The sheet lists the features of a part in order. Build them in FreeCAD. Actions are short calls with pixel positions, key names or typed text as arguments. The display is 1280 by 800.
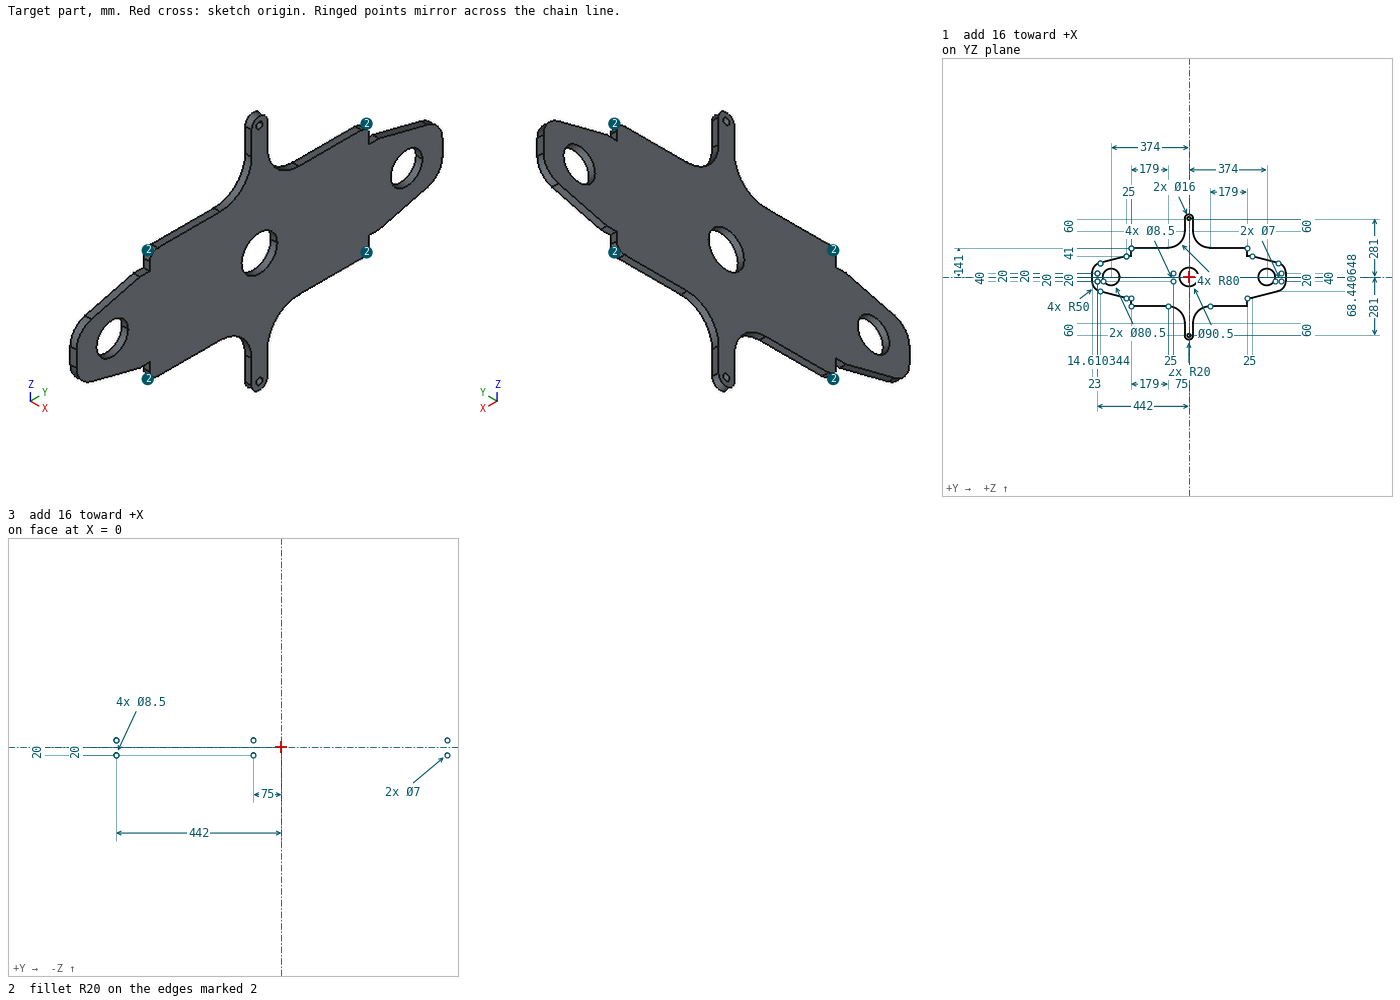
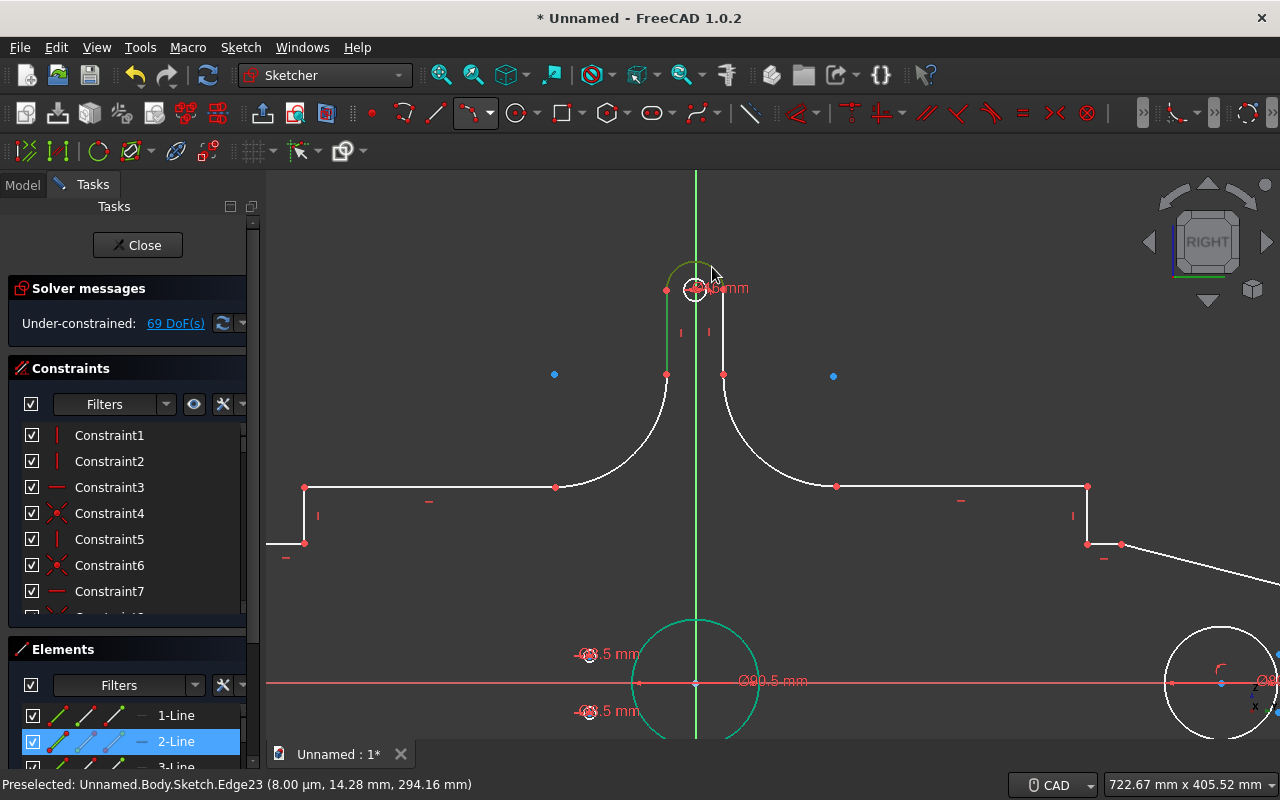
click(992, 114)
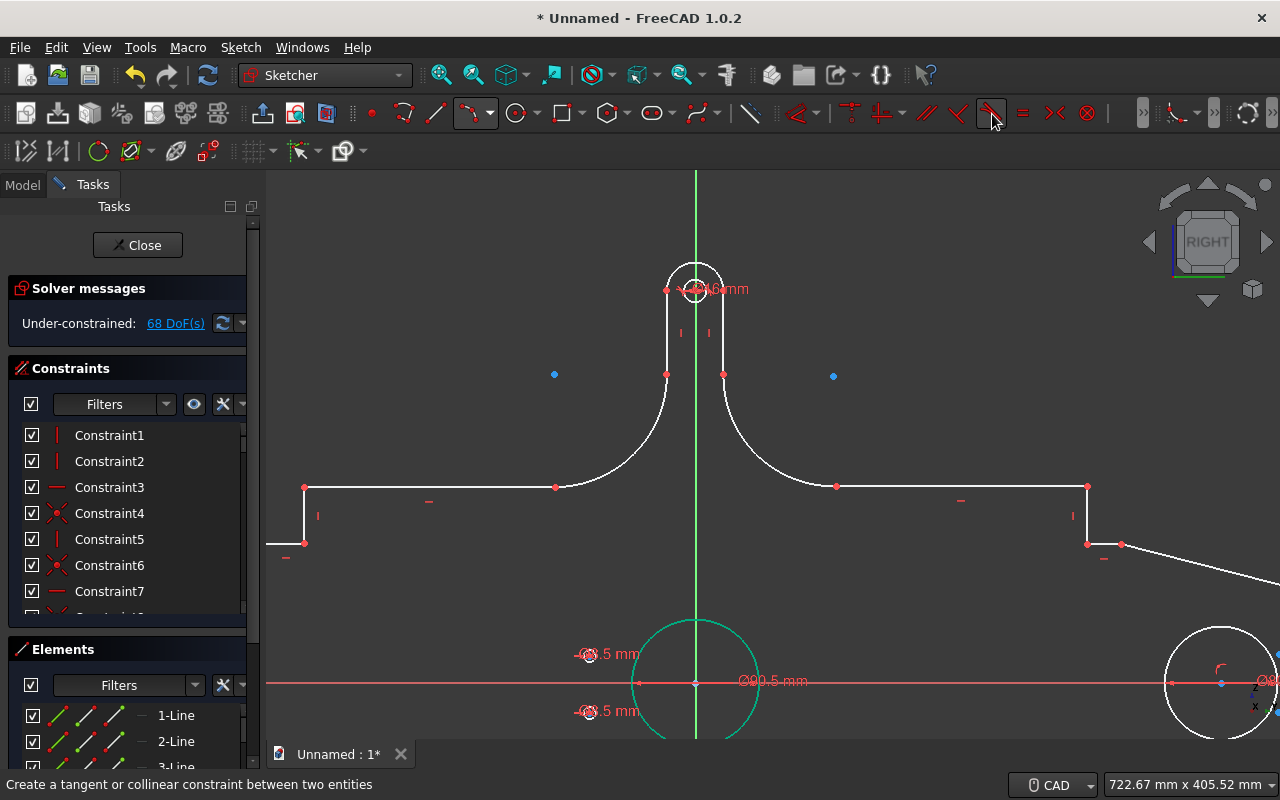
scroll(712, 268, down, 4)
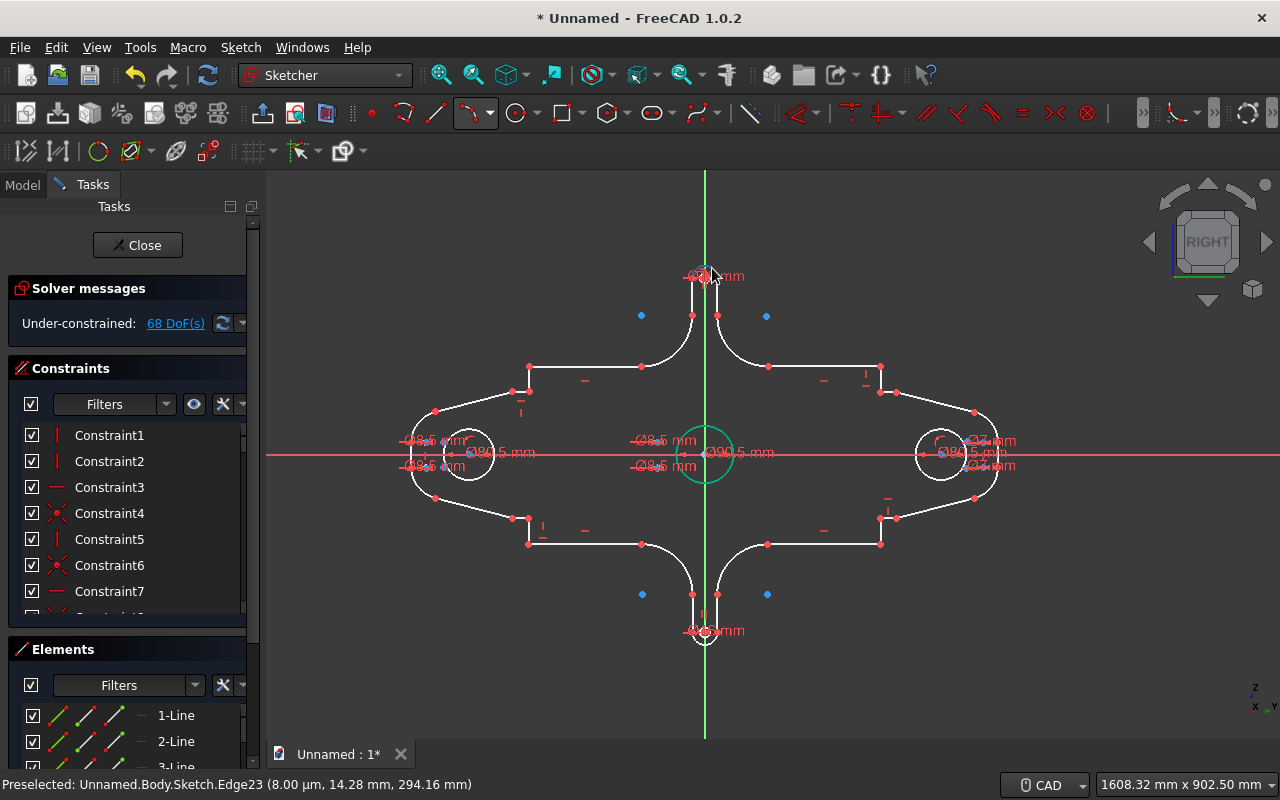
click(693, 606)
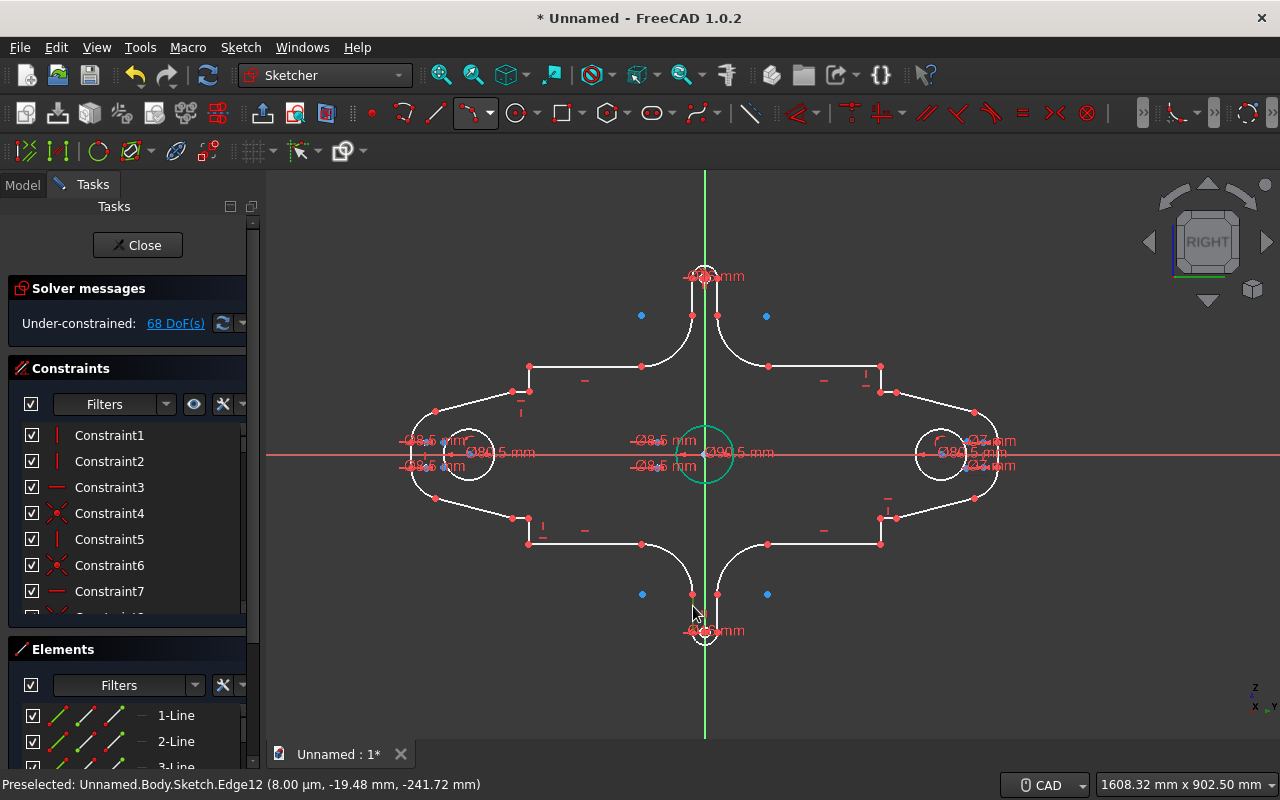
scroll(695, 640, up, 4)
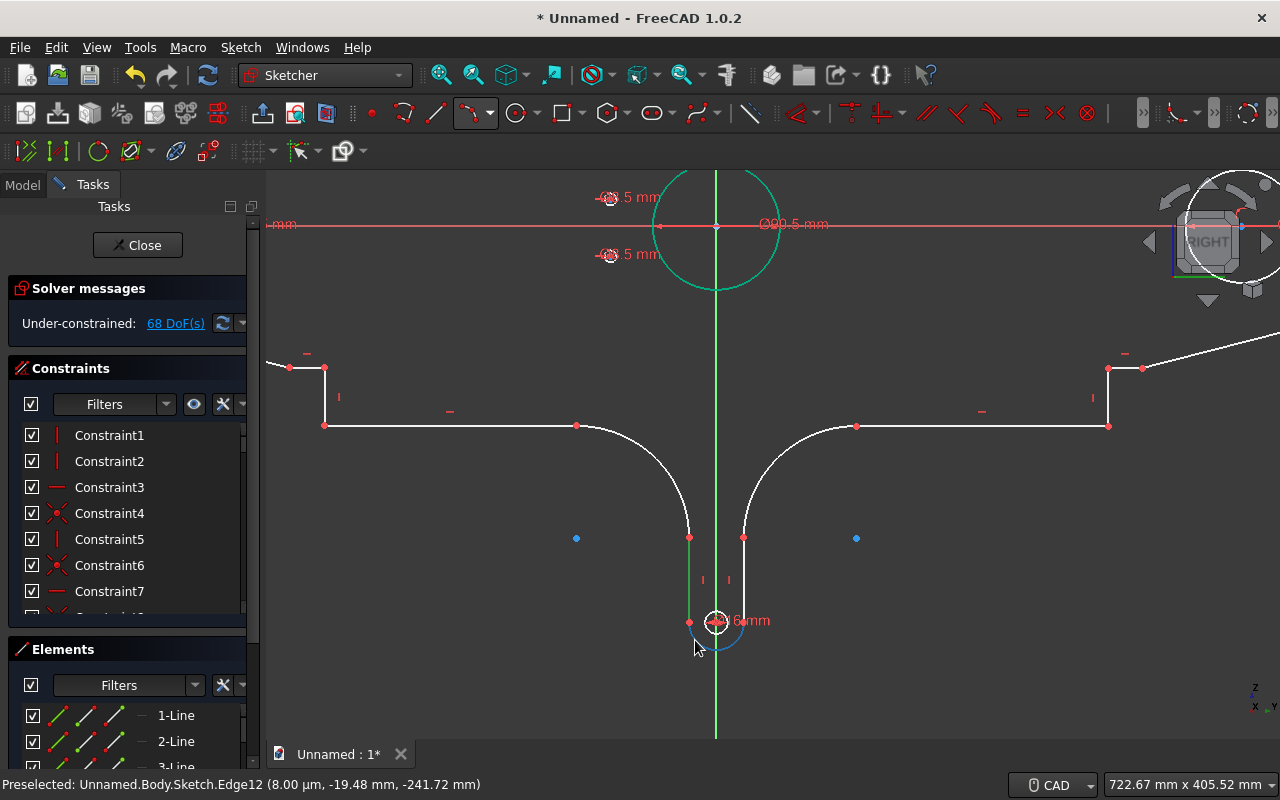
click(694, 639)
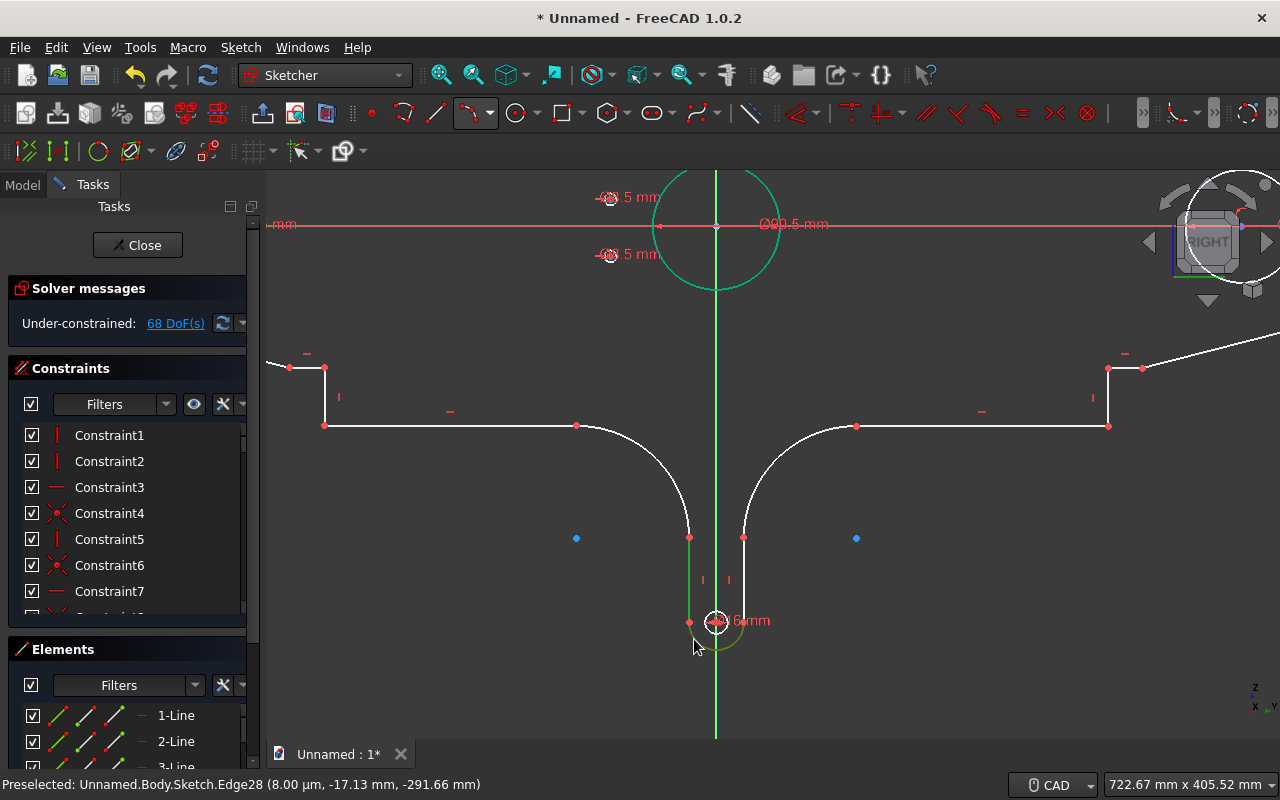
click(992, 114)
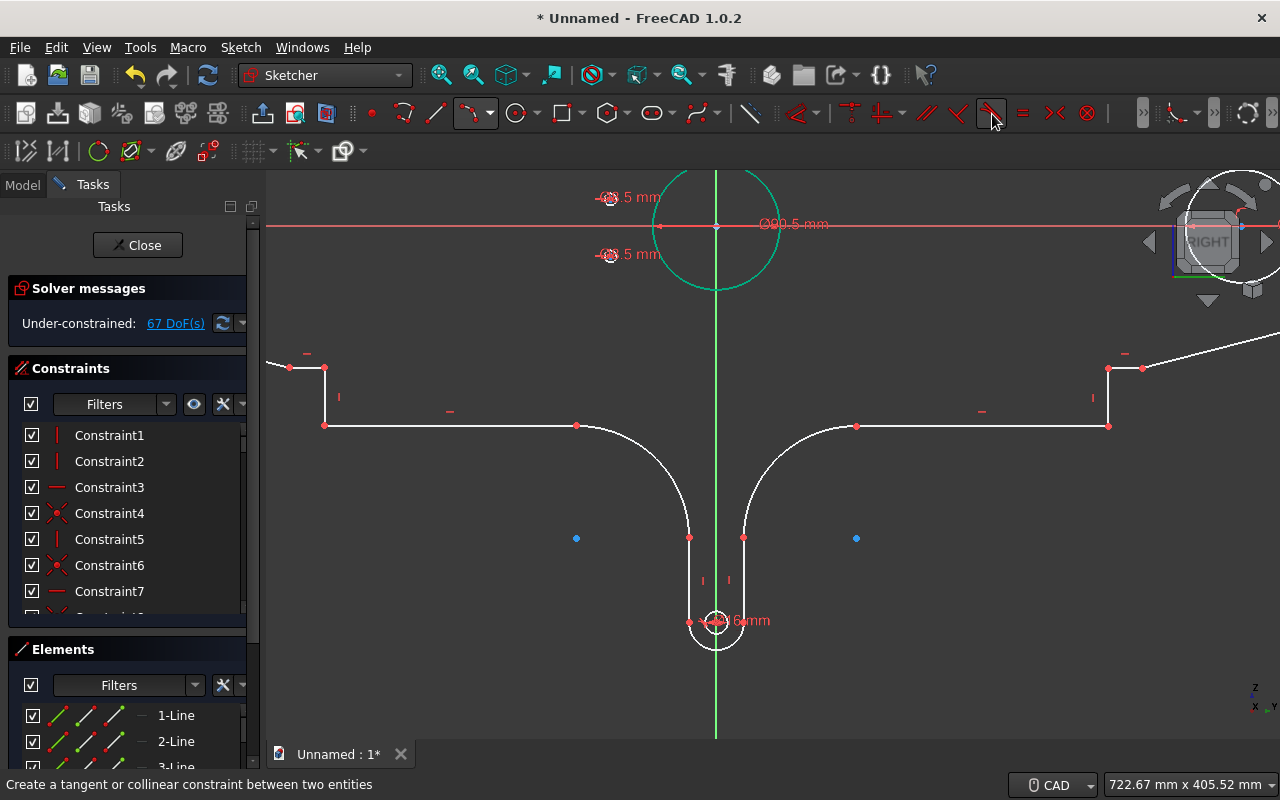
click(744, 597)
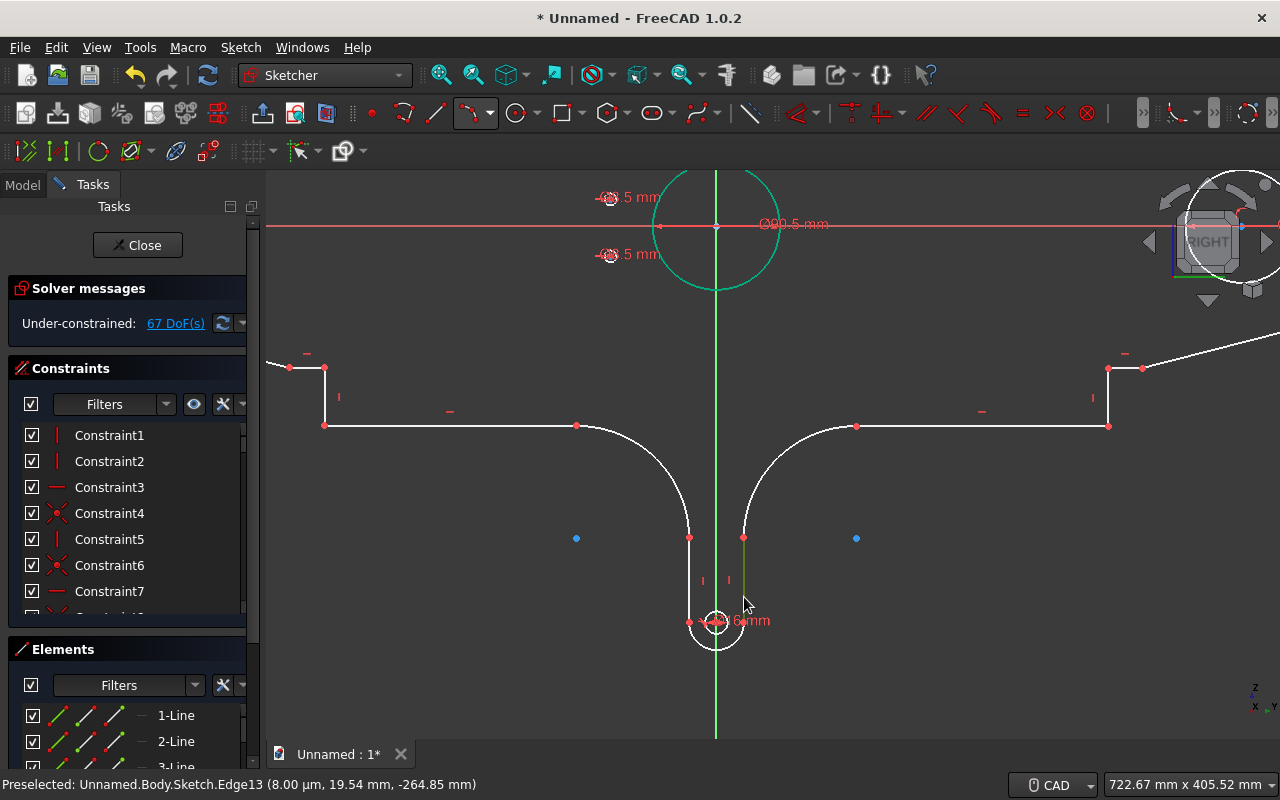
click(700, 645)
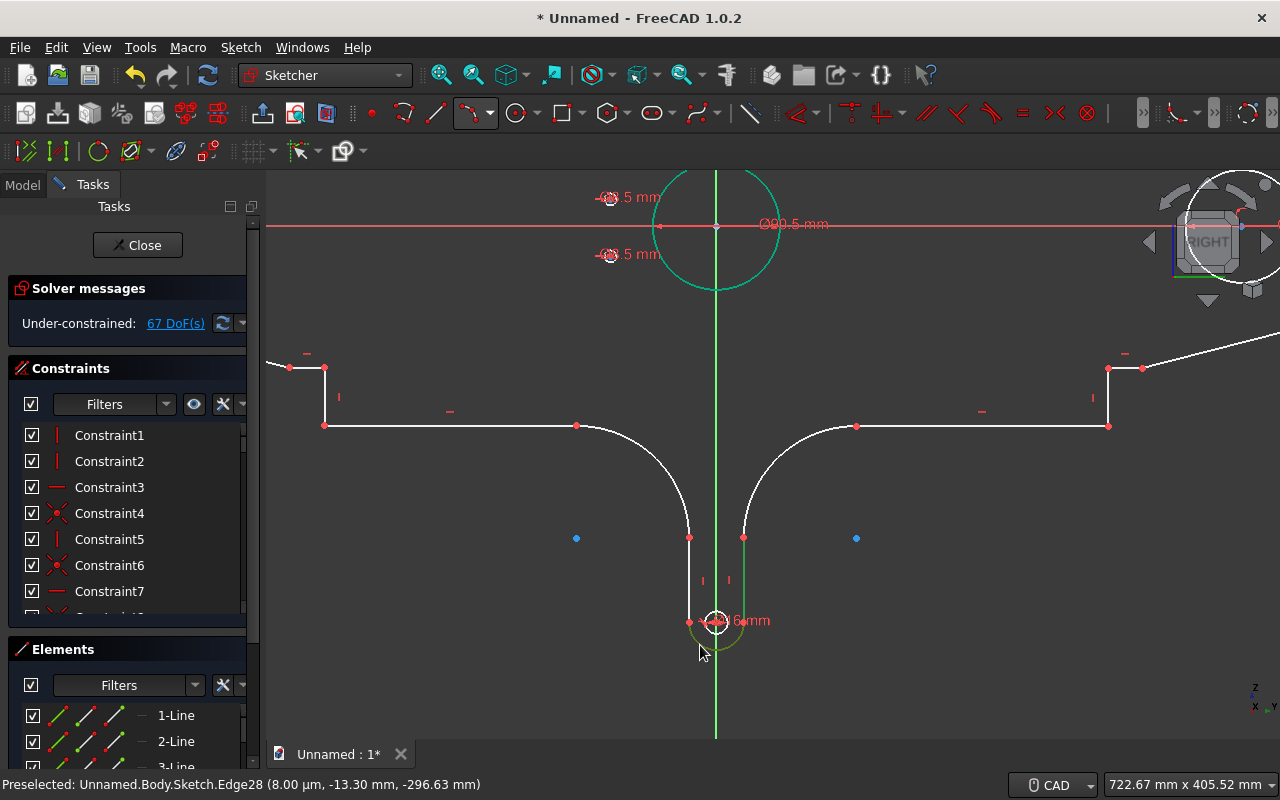
click(992, 114)